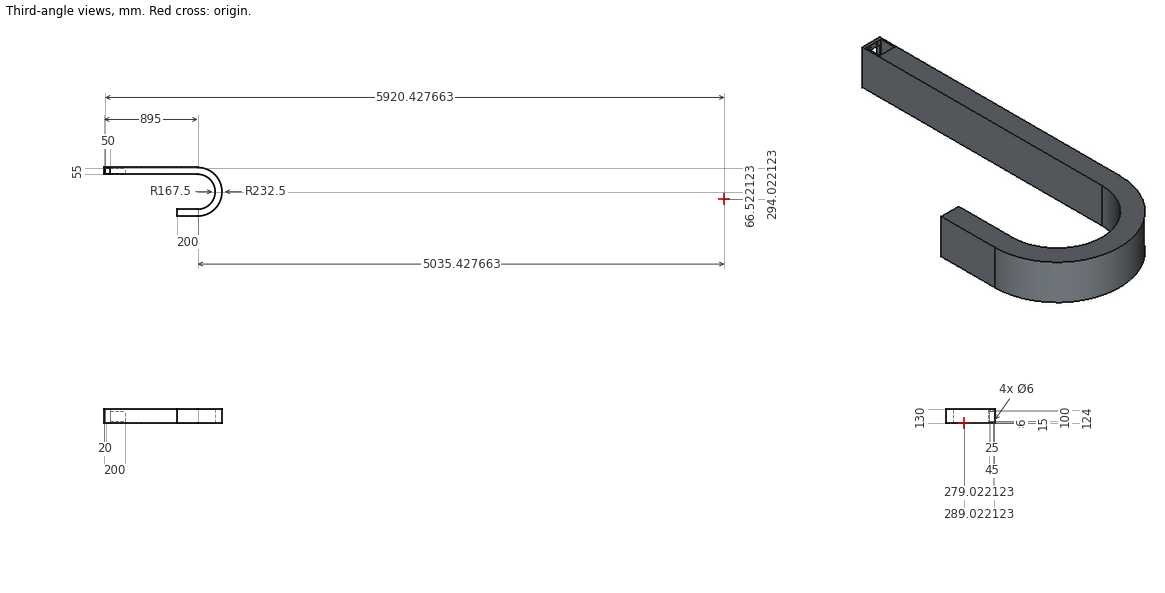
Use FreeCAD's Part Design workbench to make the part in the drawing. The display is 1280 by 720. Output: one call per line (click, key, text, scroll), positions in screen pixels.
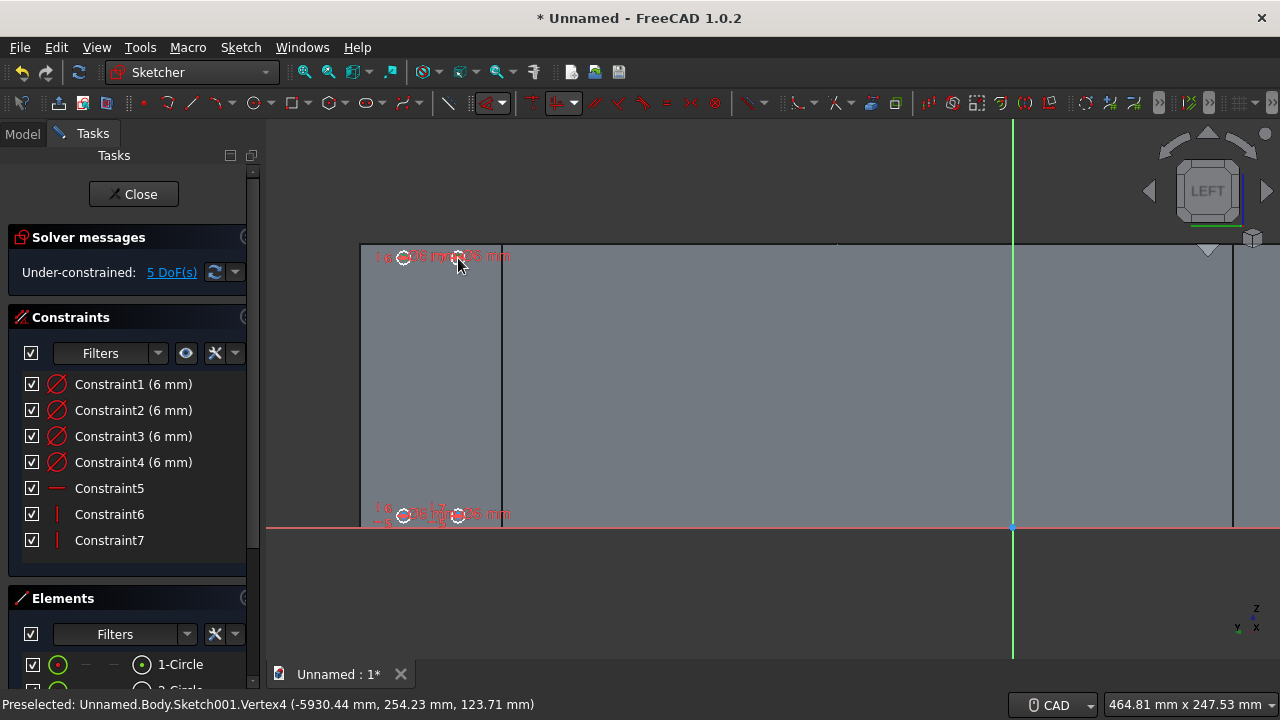
key(h)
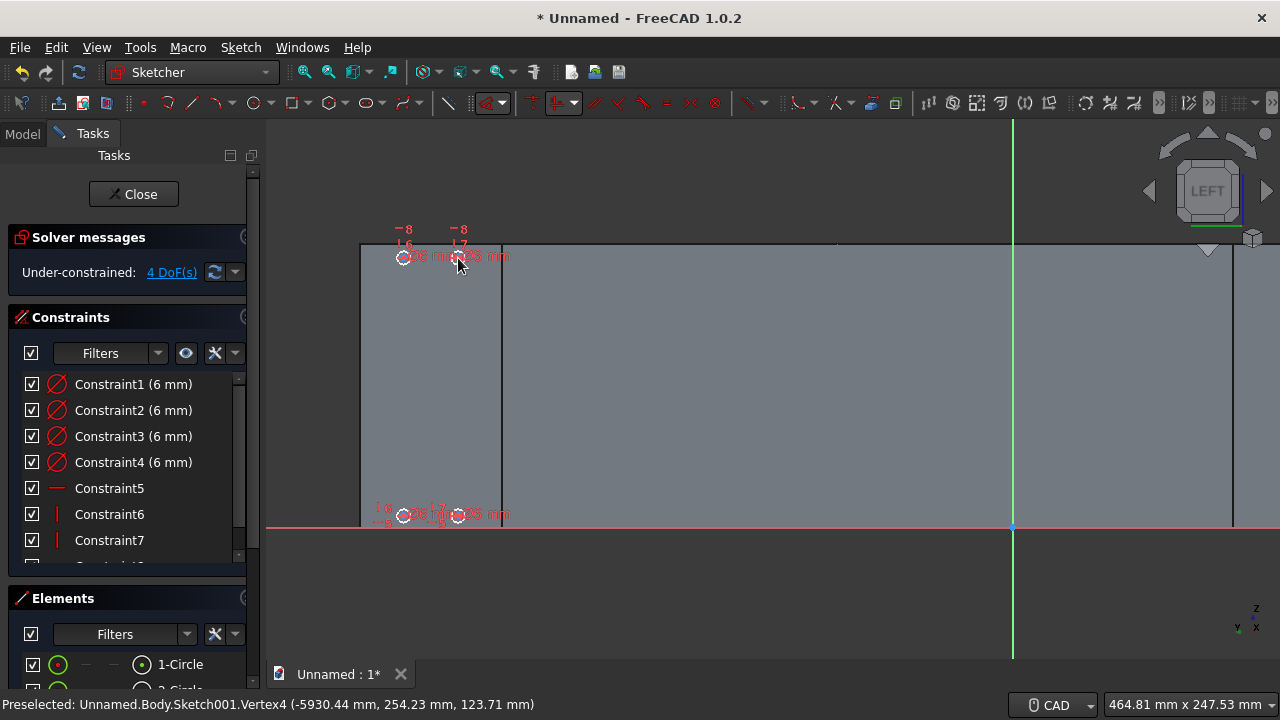
scroll(404, 516, up, 6)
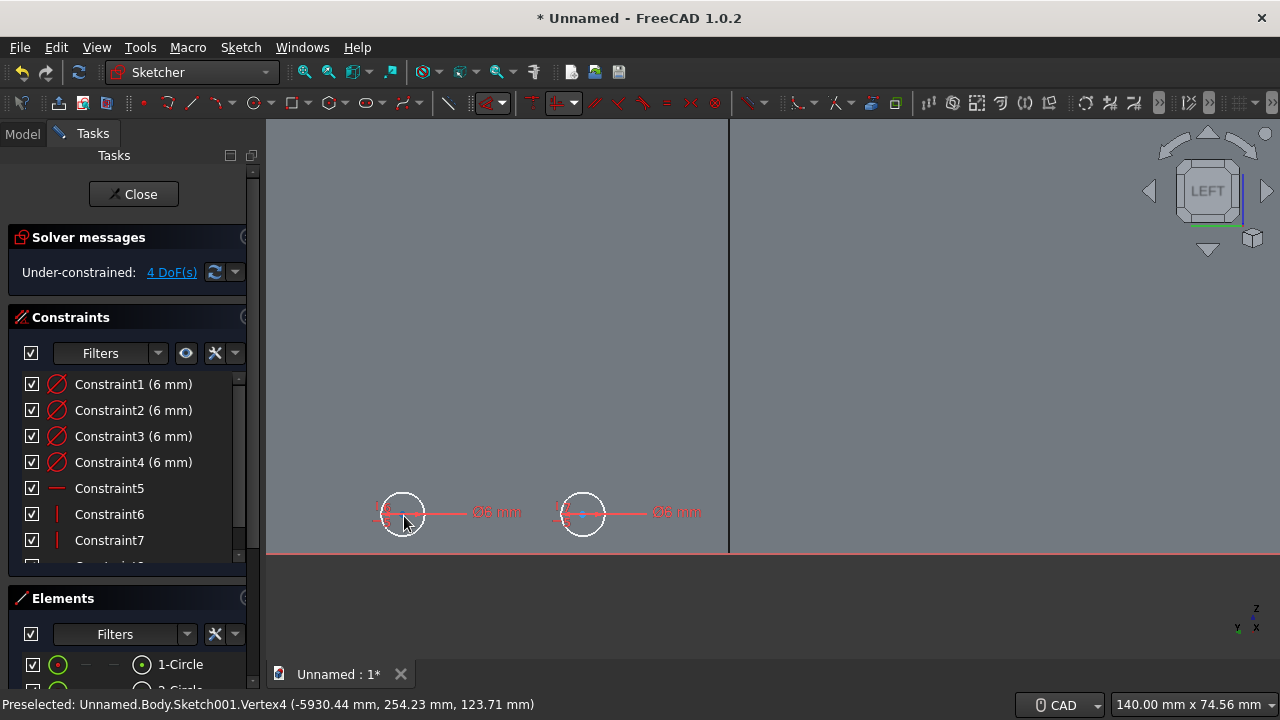
click(403, 514)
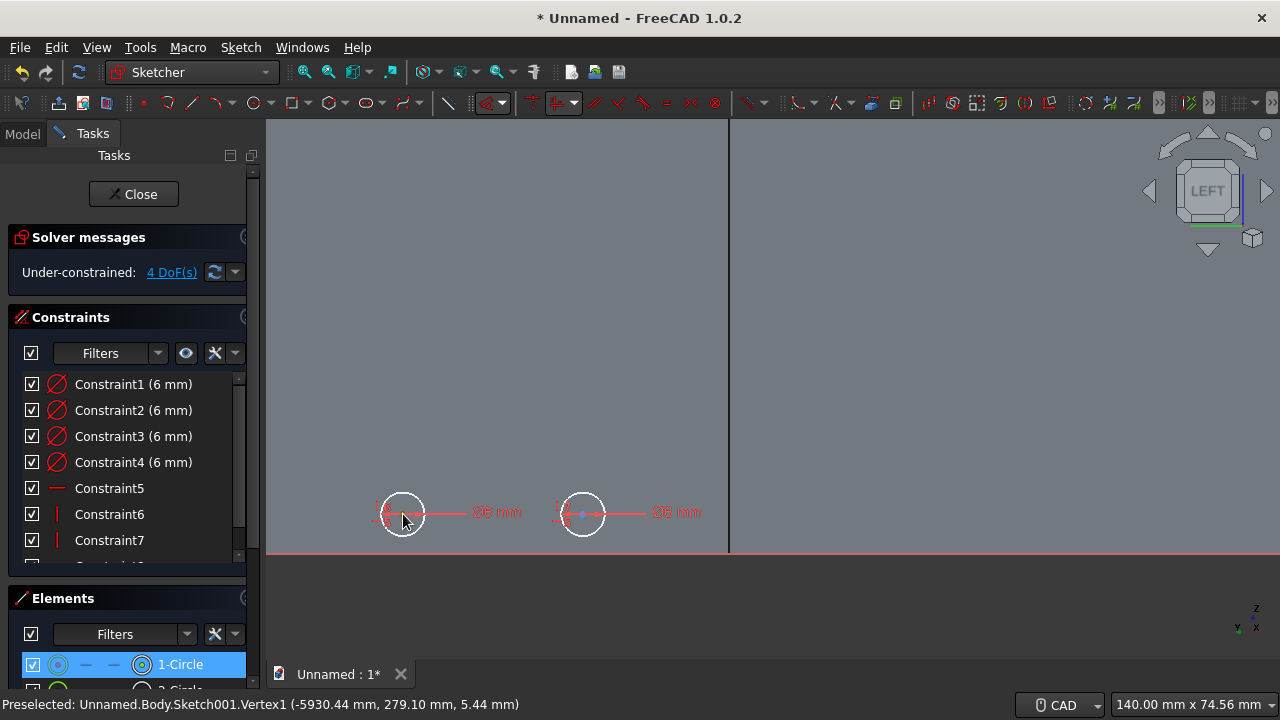
key(i)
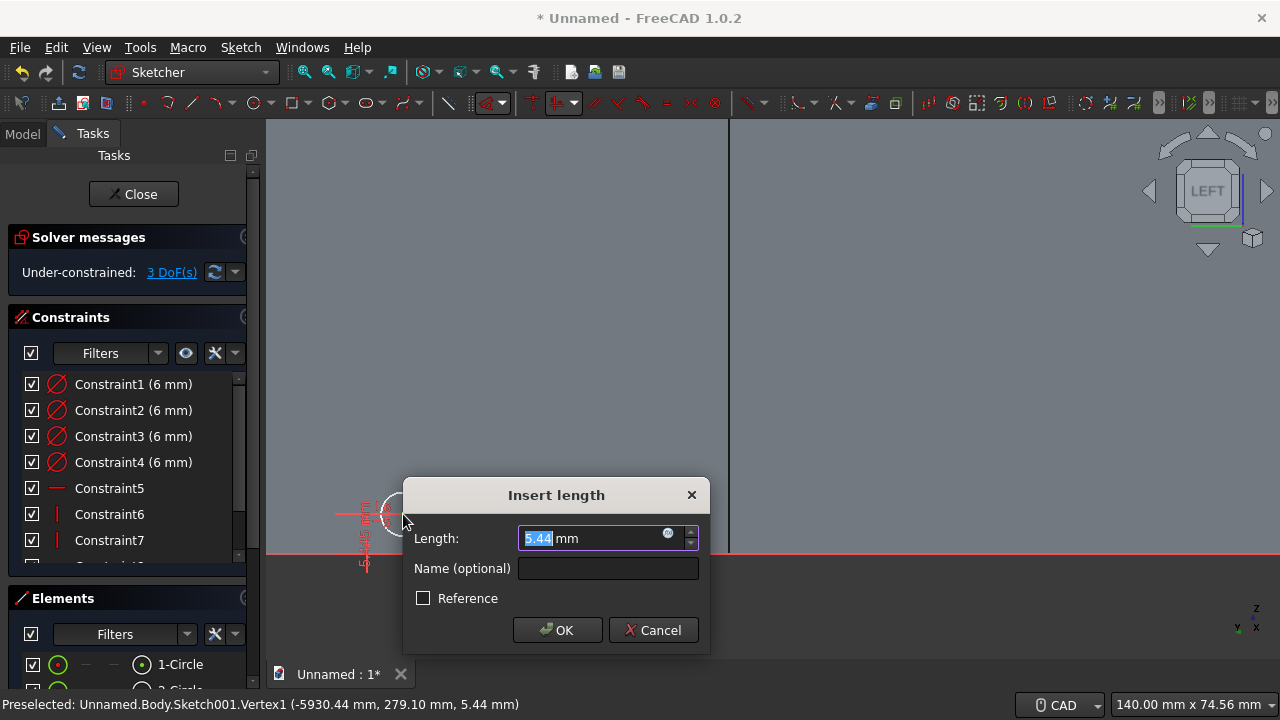
text(6)
key(Return)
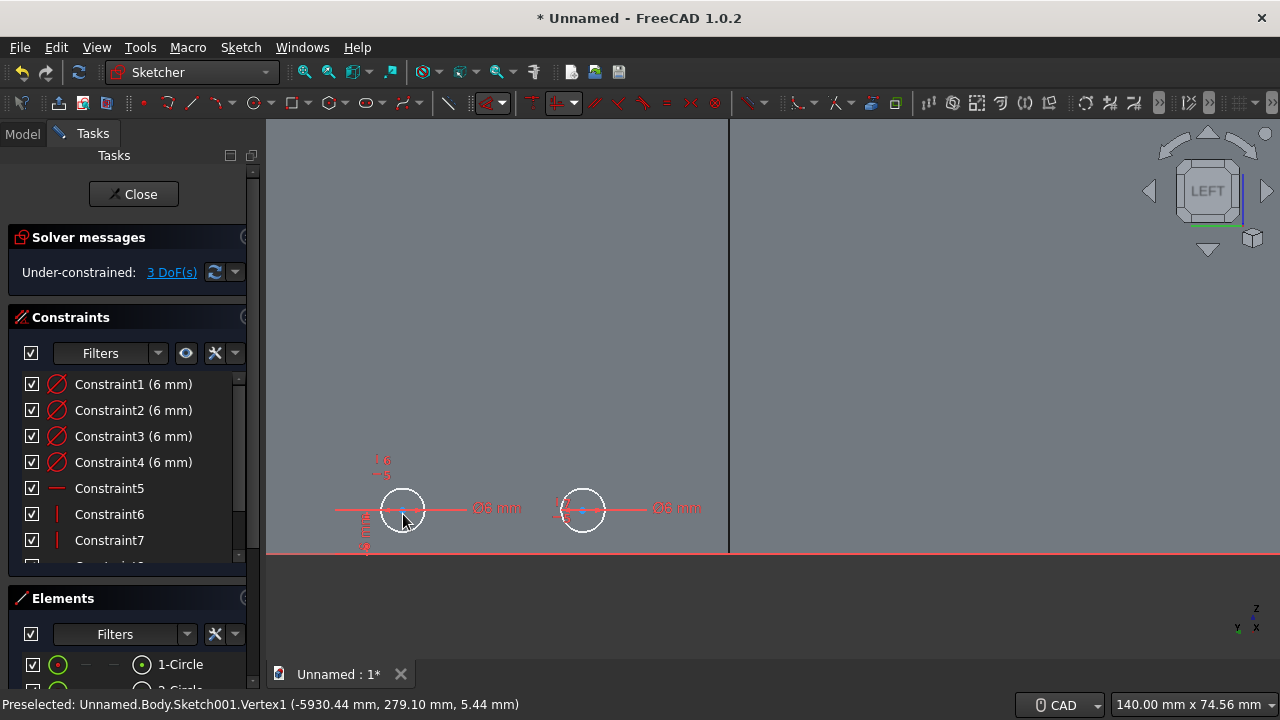
scroll(403, 516, down, 6)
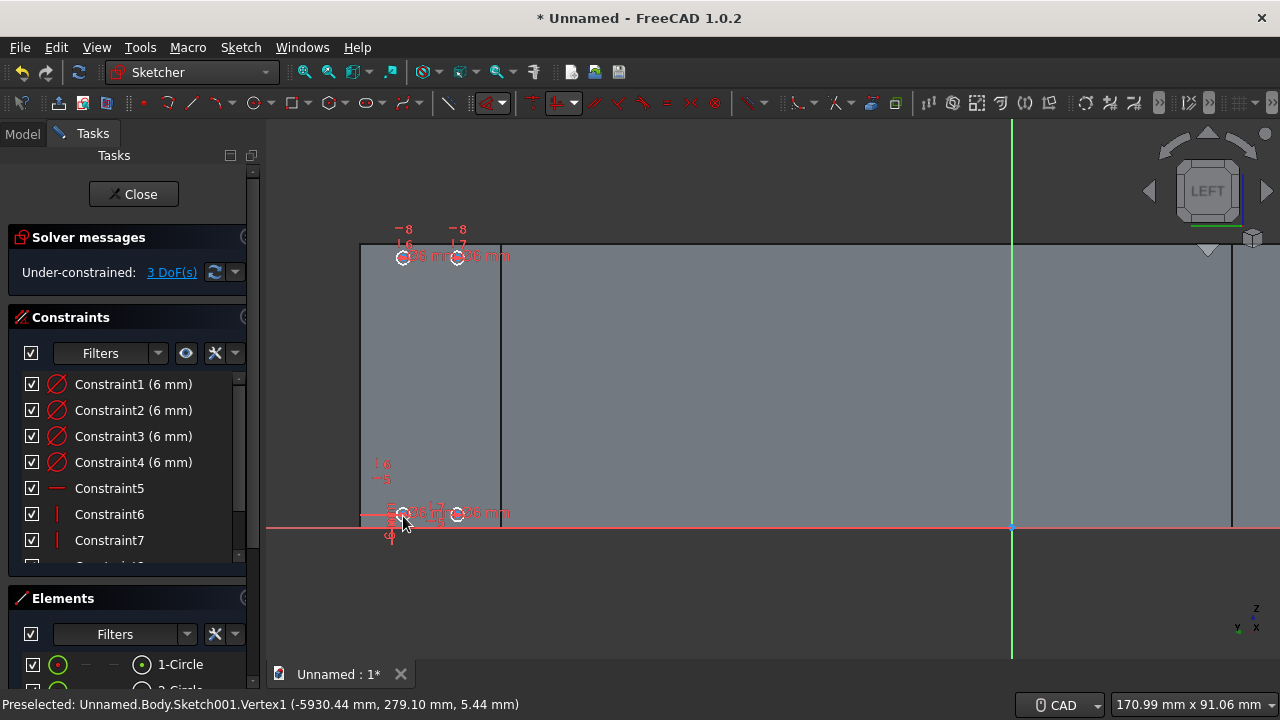
click(403, 258)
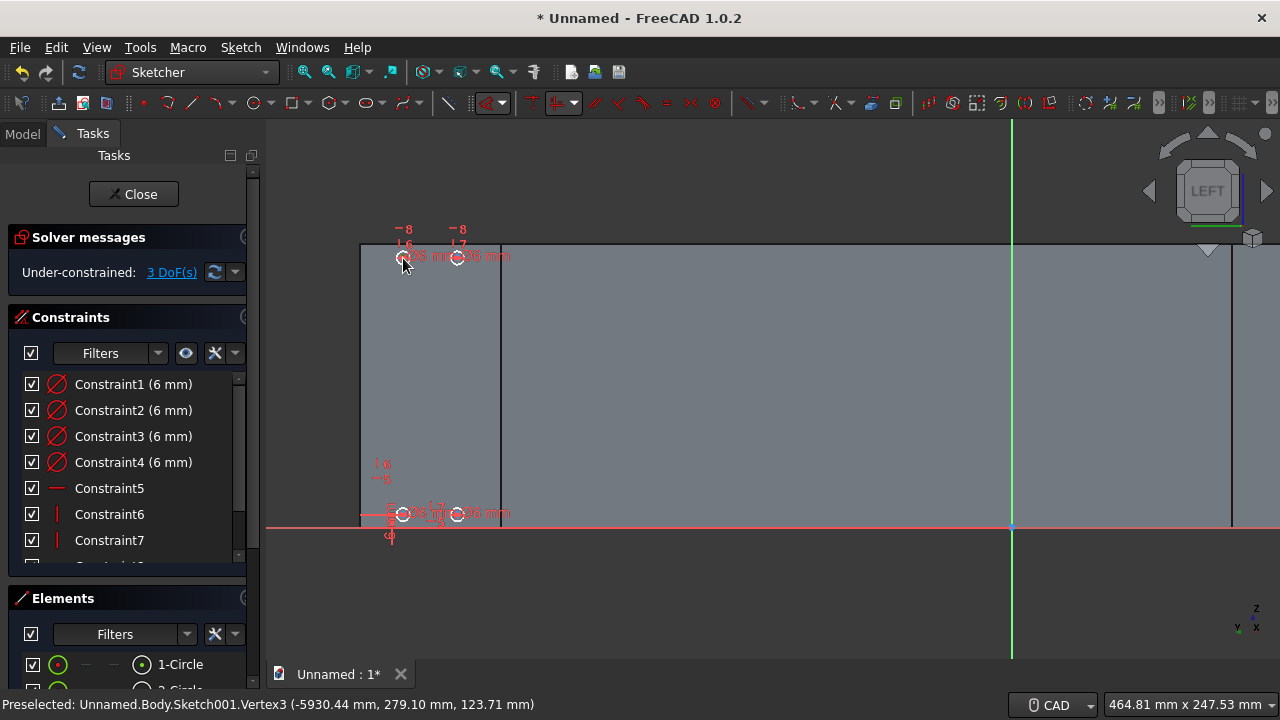
click(504, 104)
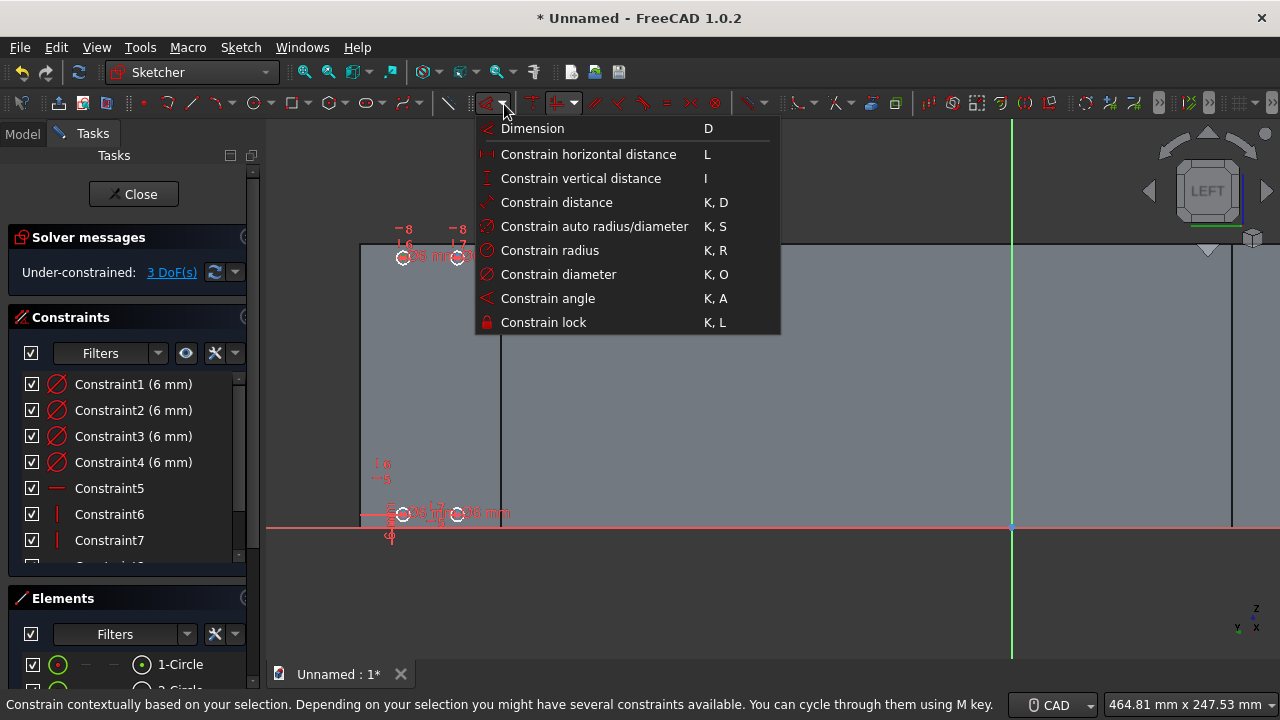
click(628, 178)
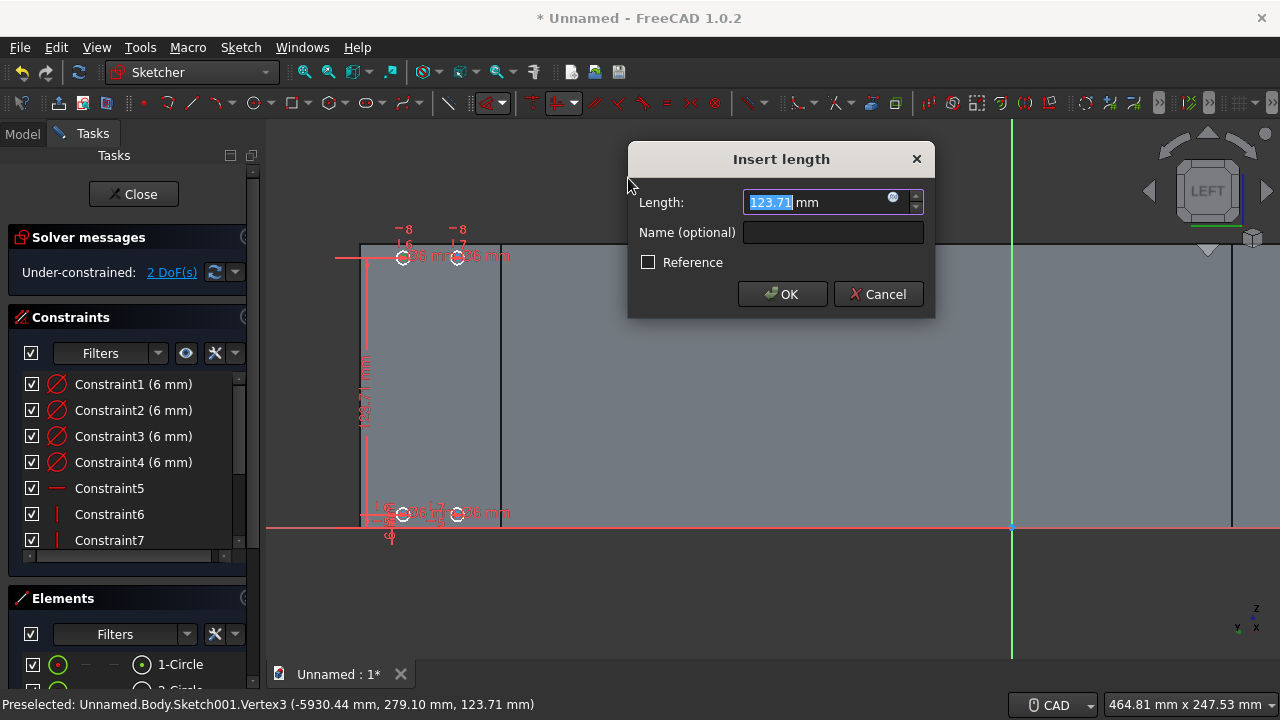
text(124)
key(Return)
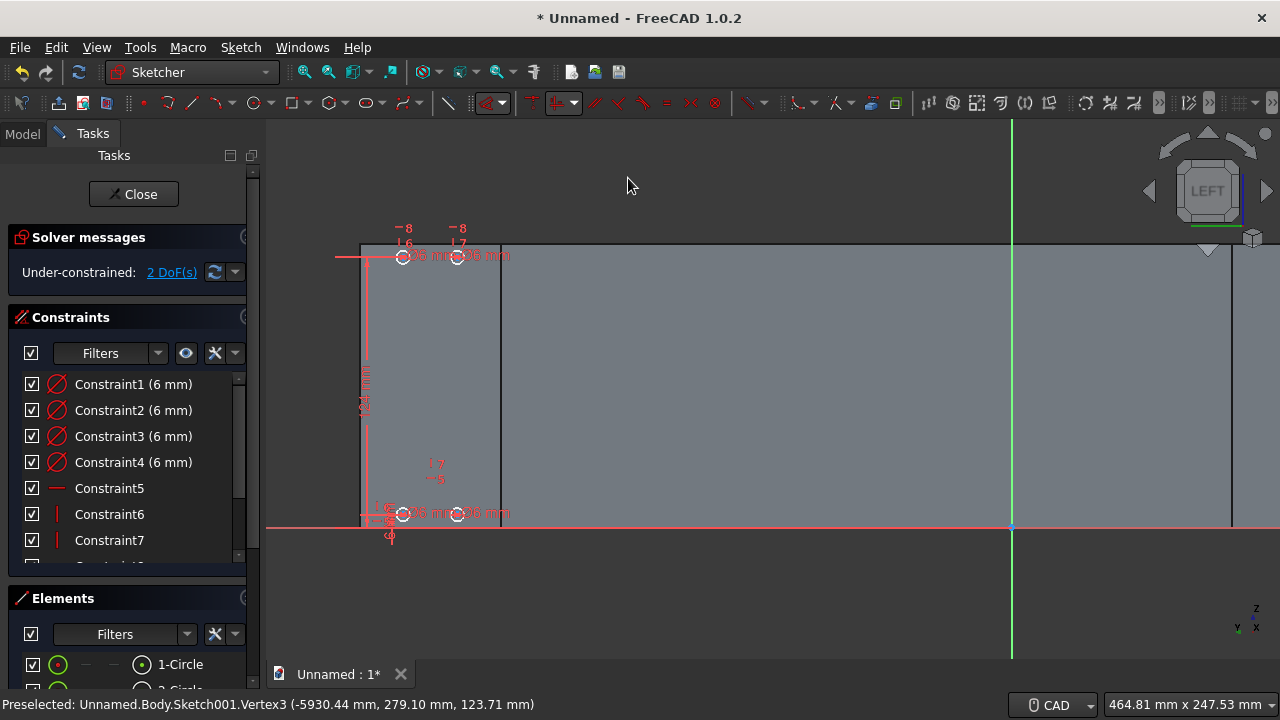
click(403, 515)